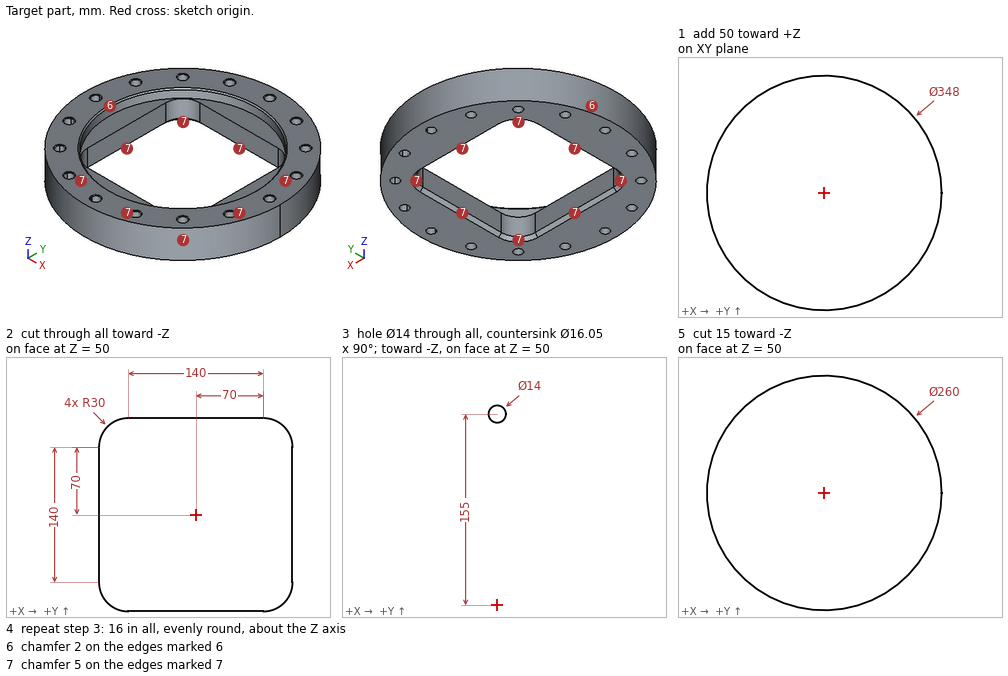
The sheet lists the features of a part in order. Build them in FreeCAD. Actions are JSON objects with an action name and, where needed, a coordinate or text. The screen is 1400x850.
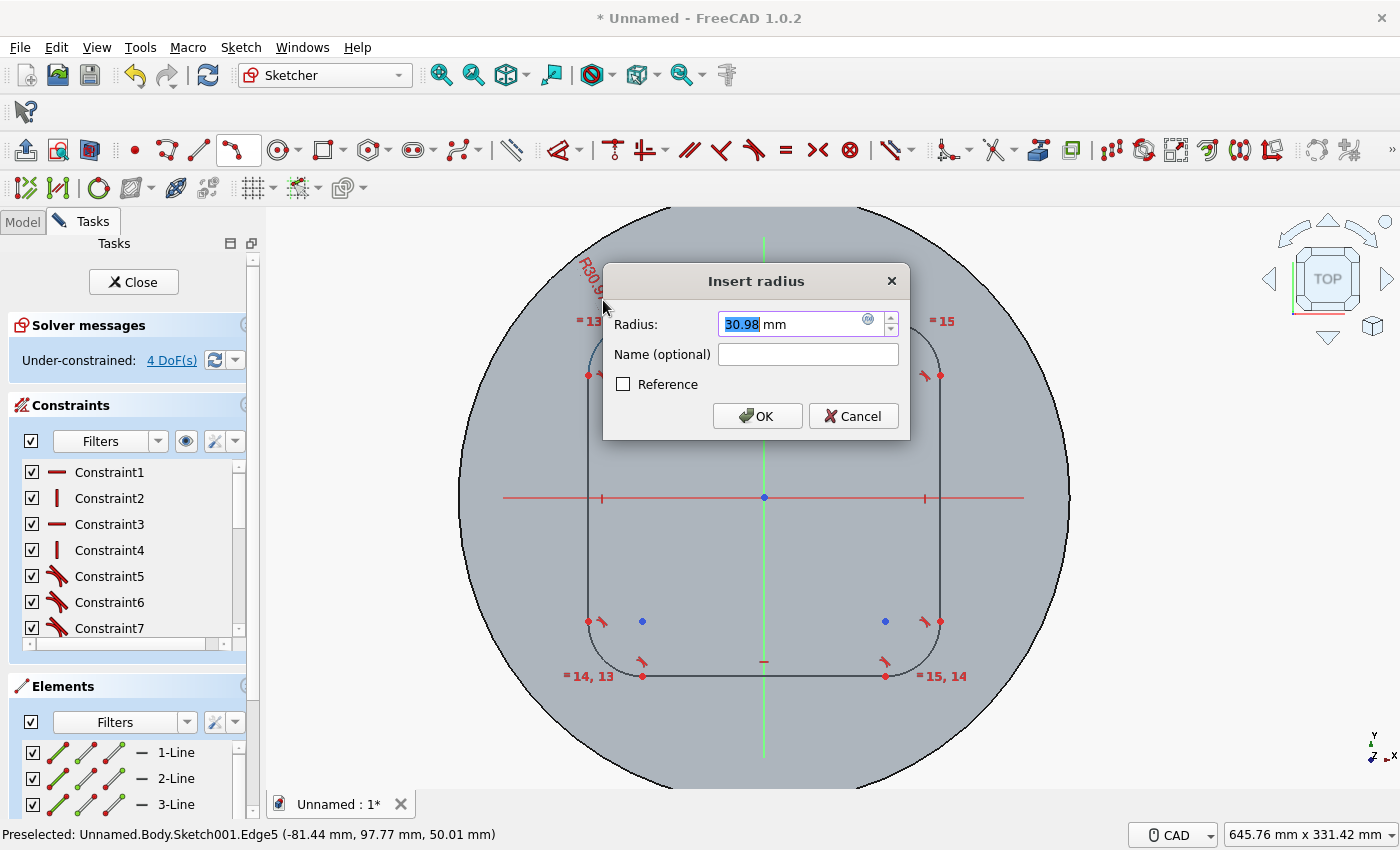
{"action": "type", "text": "30"}
{"action": "key", "text": "Return"}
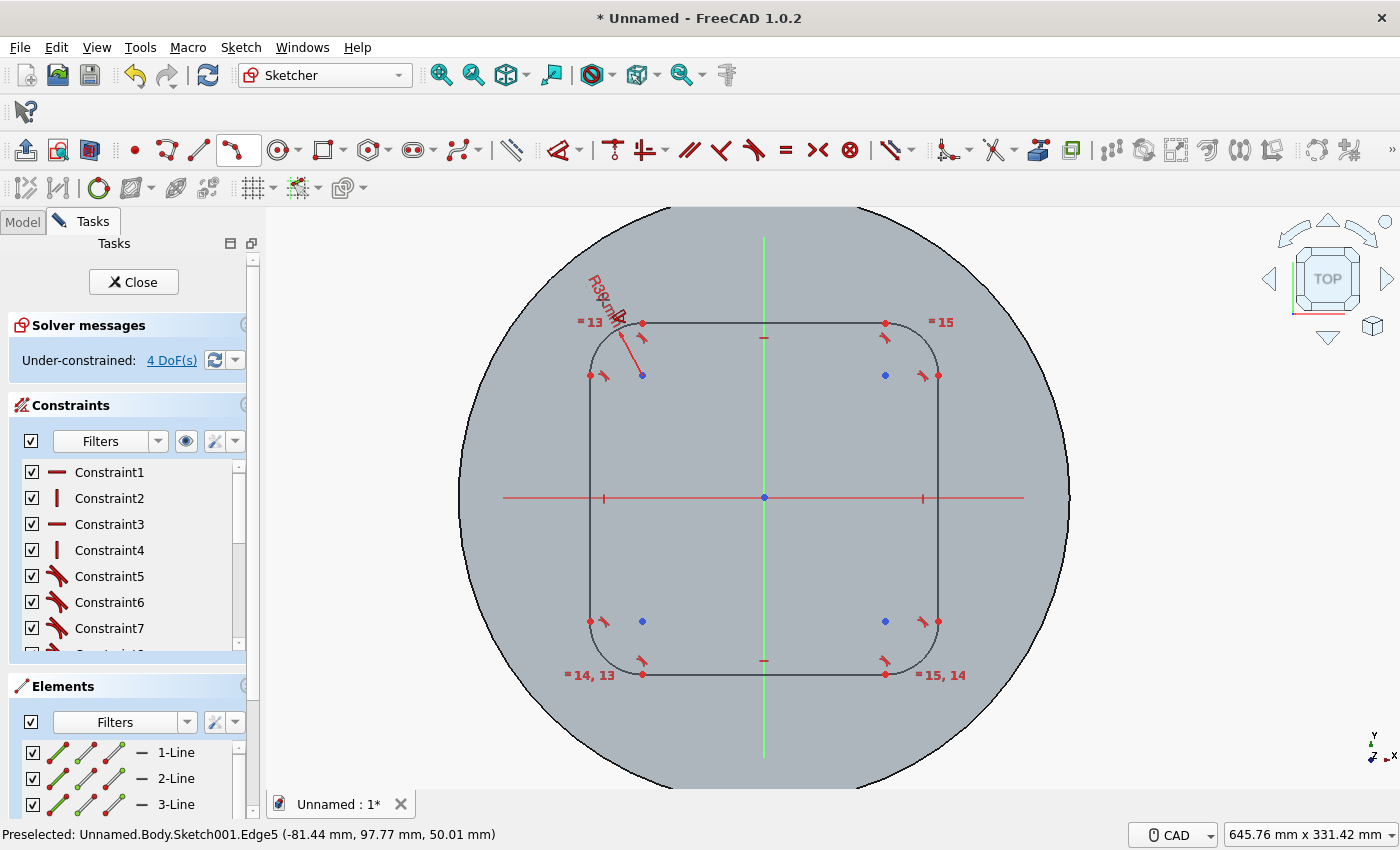
{"action": "left_click", "coordinate": [813, 323]}
{"action": "left_click", "coordinate": [708, 289]}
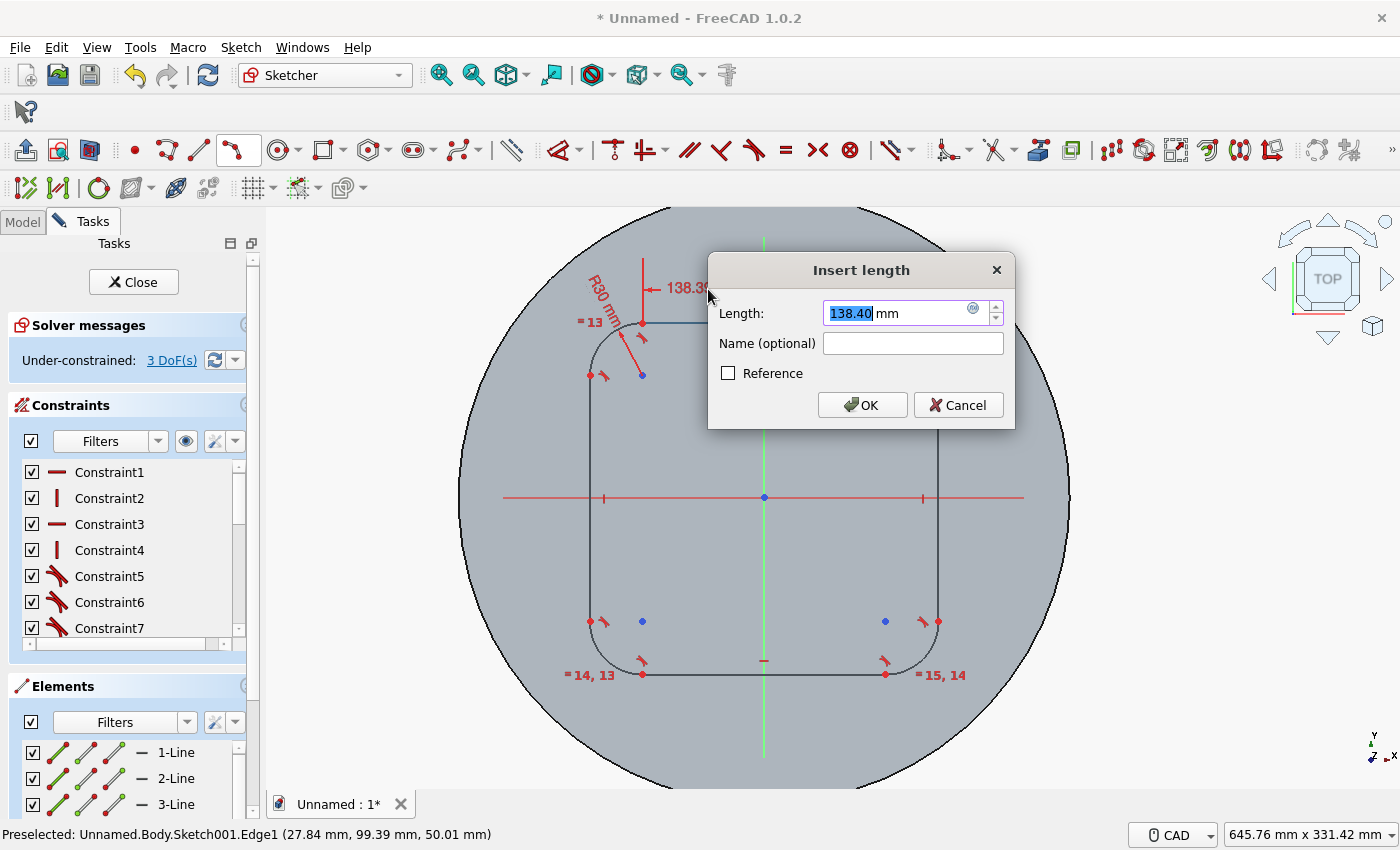
{"action": "type", "text": "140"}
{"action": "key", "text": "Return"}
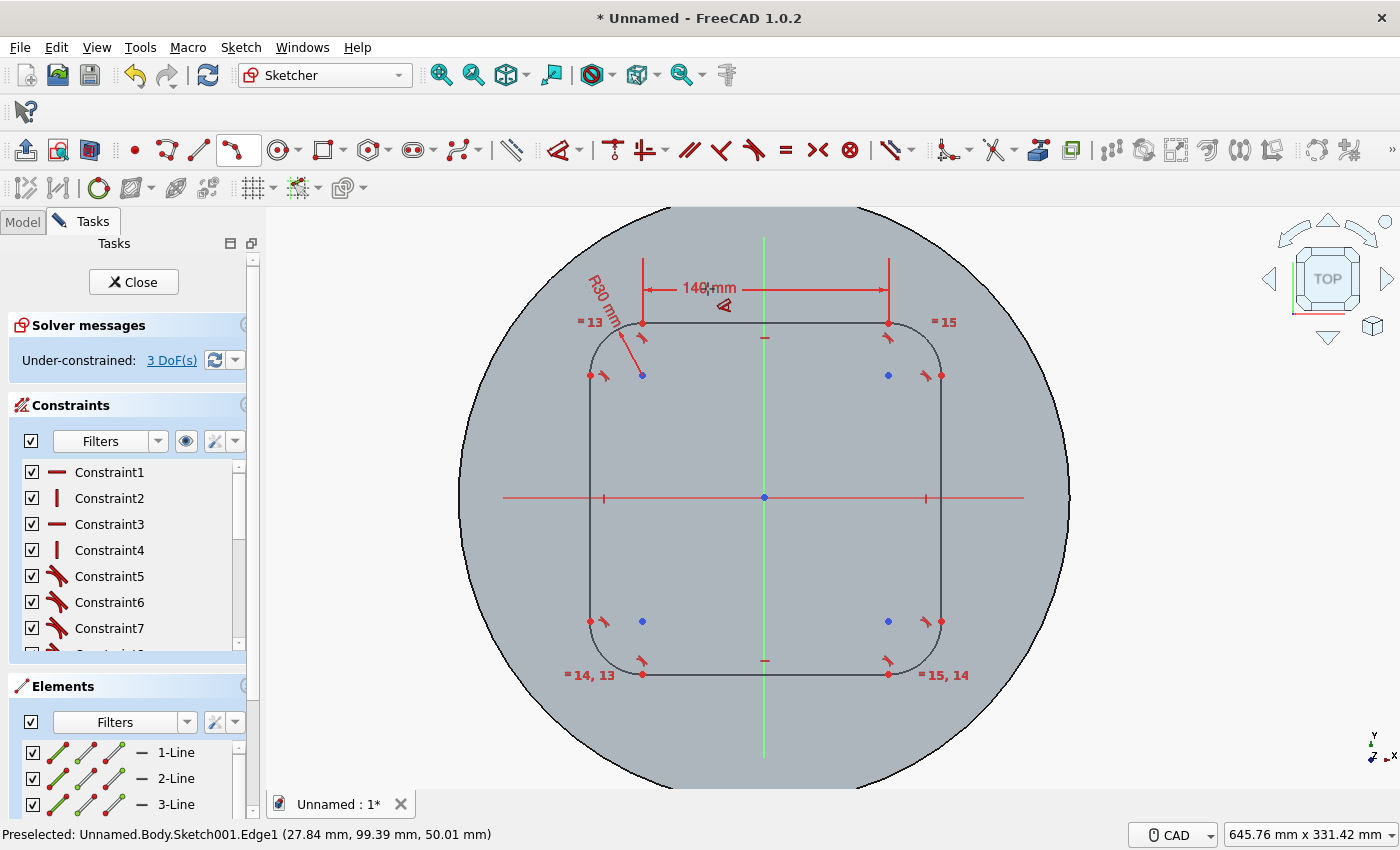
{"action": "left_click", "coordinate": [590, 450]}
{"action": "left_click", "coordinate": [556, 442]}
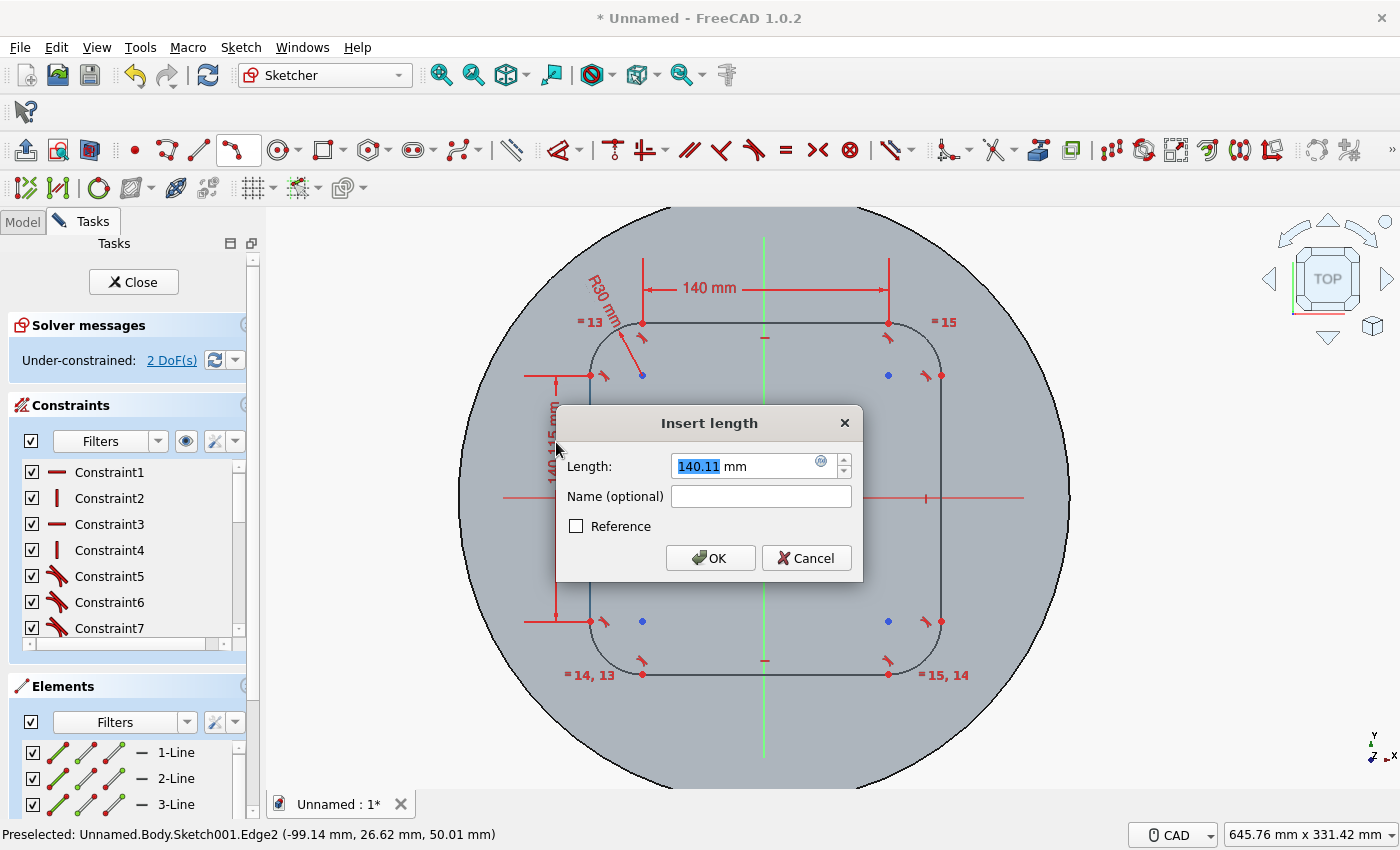
{"action": "type", "text": "140"}
{"action": "key", "text": "Return"}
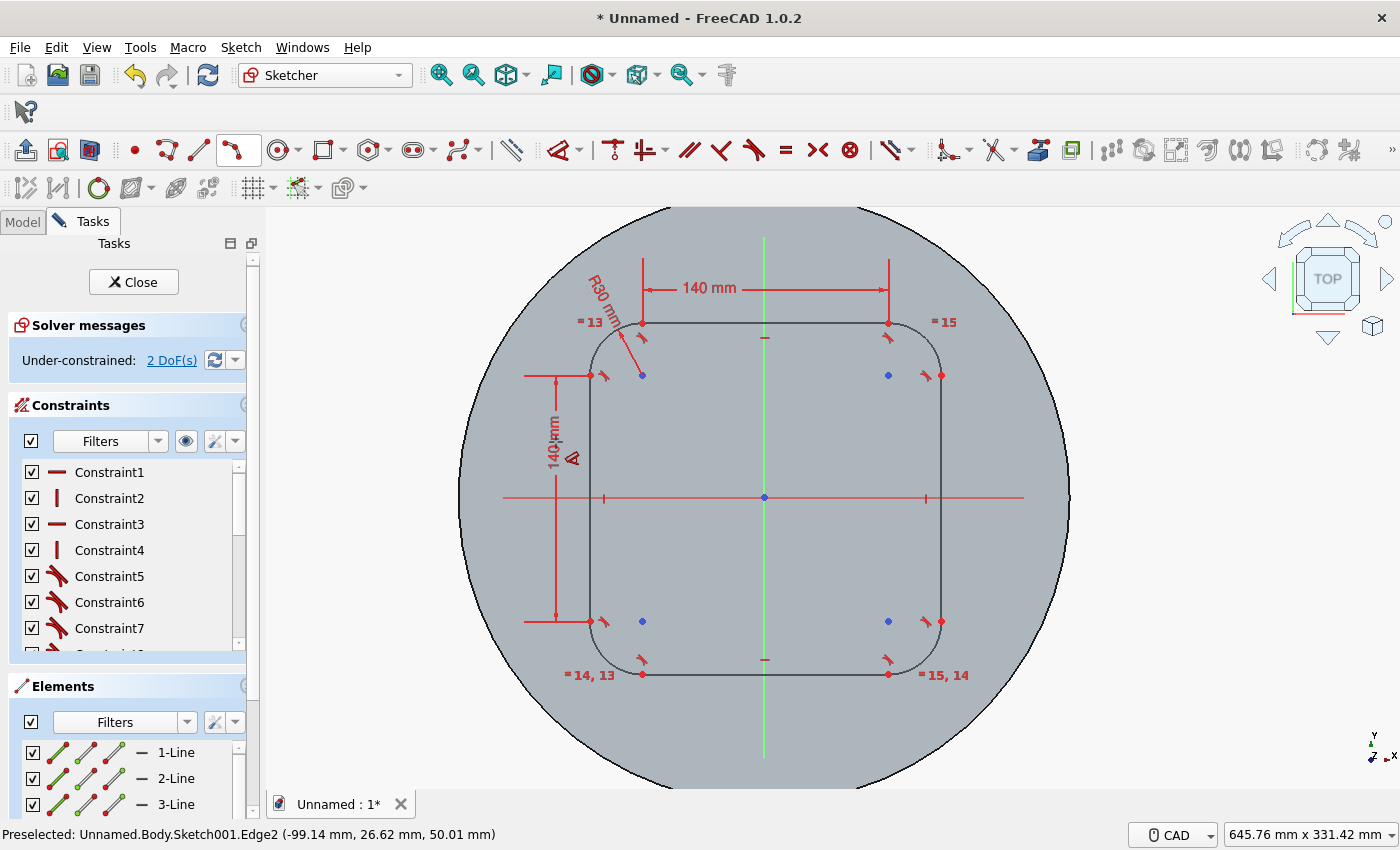
{"action": "left_click", "coordinate": [889, 323]}
{"action": "left_click", "coordinate": [826, 289]}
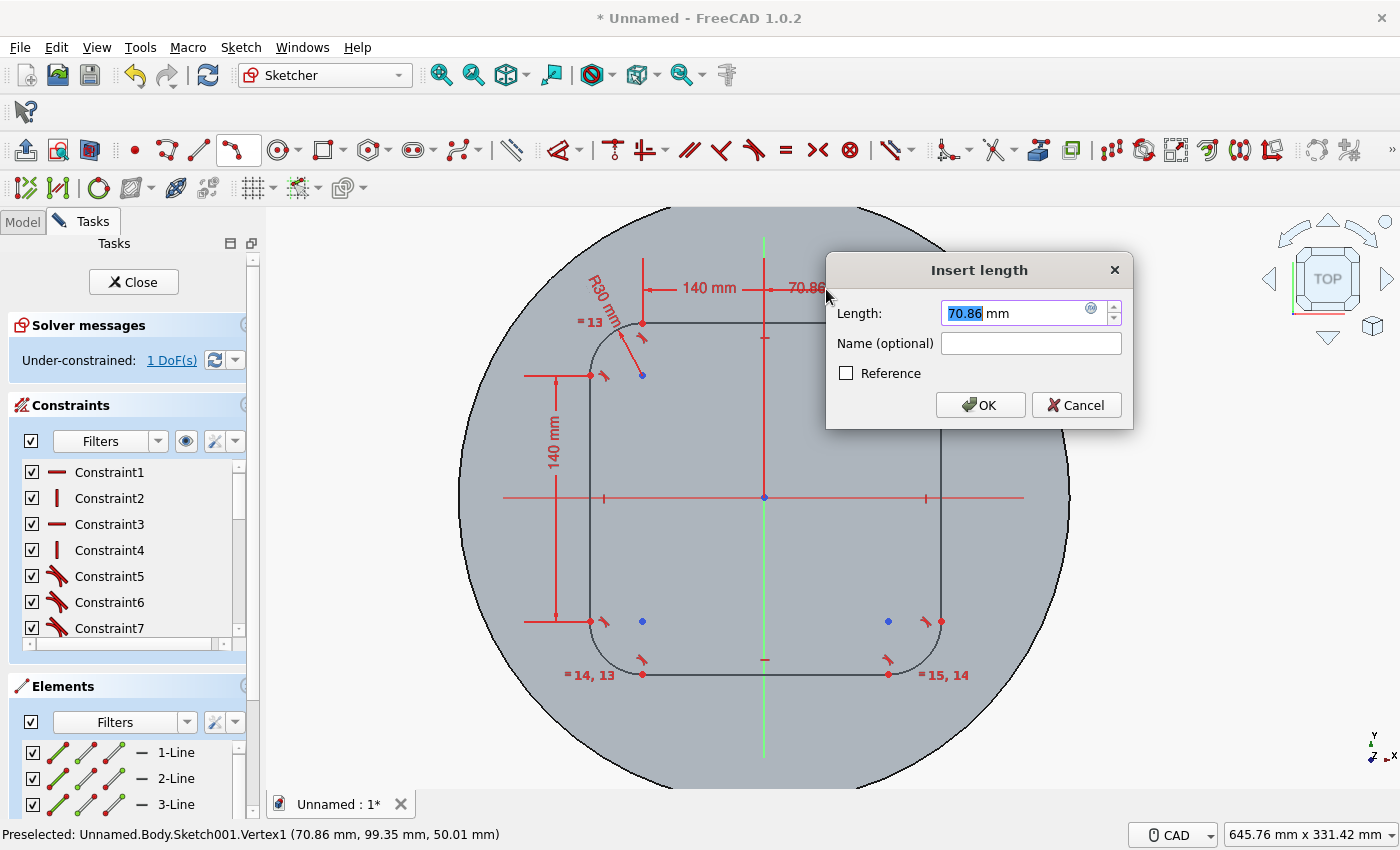
{"action": "type", "text": "70"}
{"action": "key", "text": "Return"}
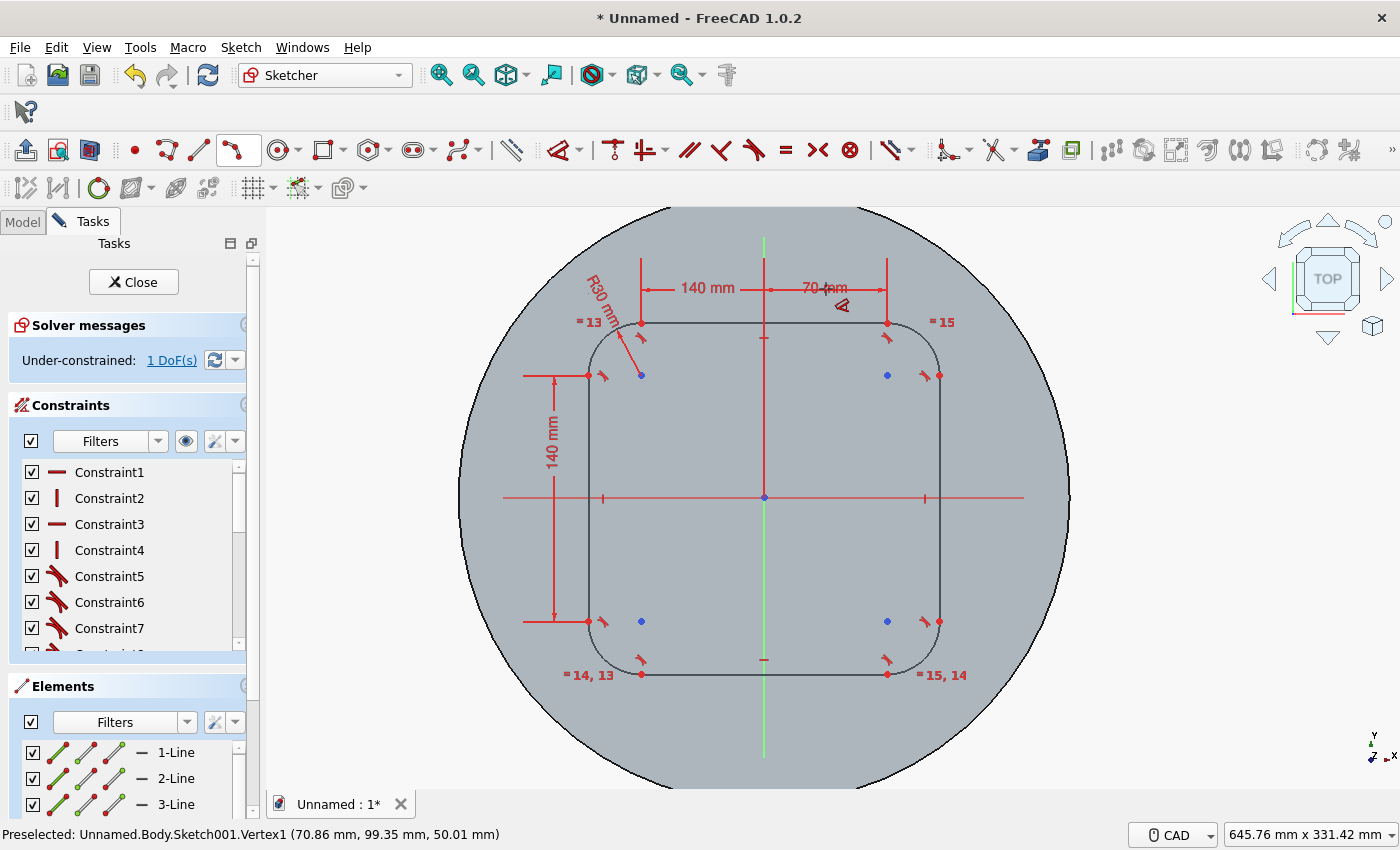
{"action": "left_click", "coordinate": [589, 376]}
{"action": "left_click", "coordinate": [555, 409]}